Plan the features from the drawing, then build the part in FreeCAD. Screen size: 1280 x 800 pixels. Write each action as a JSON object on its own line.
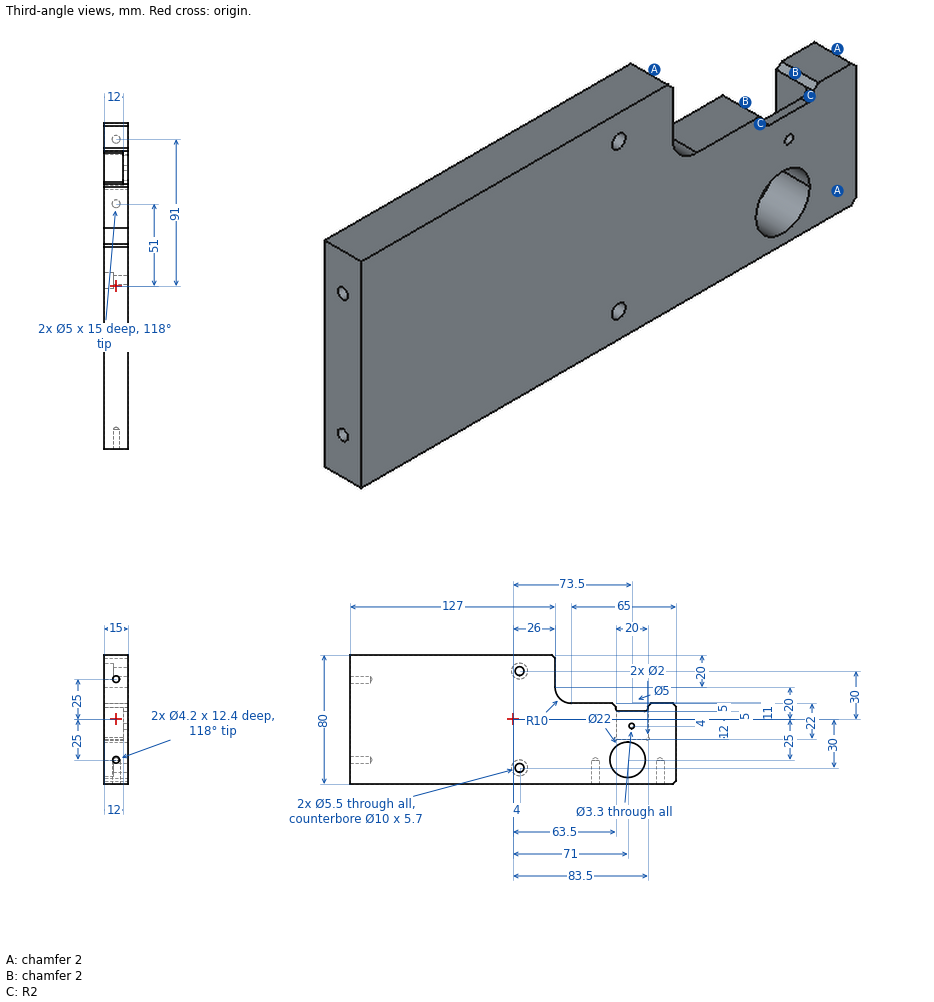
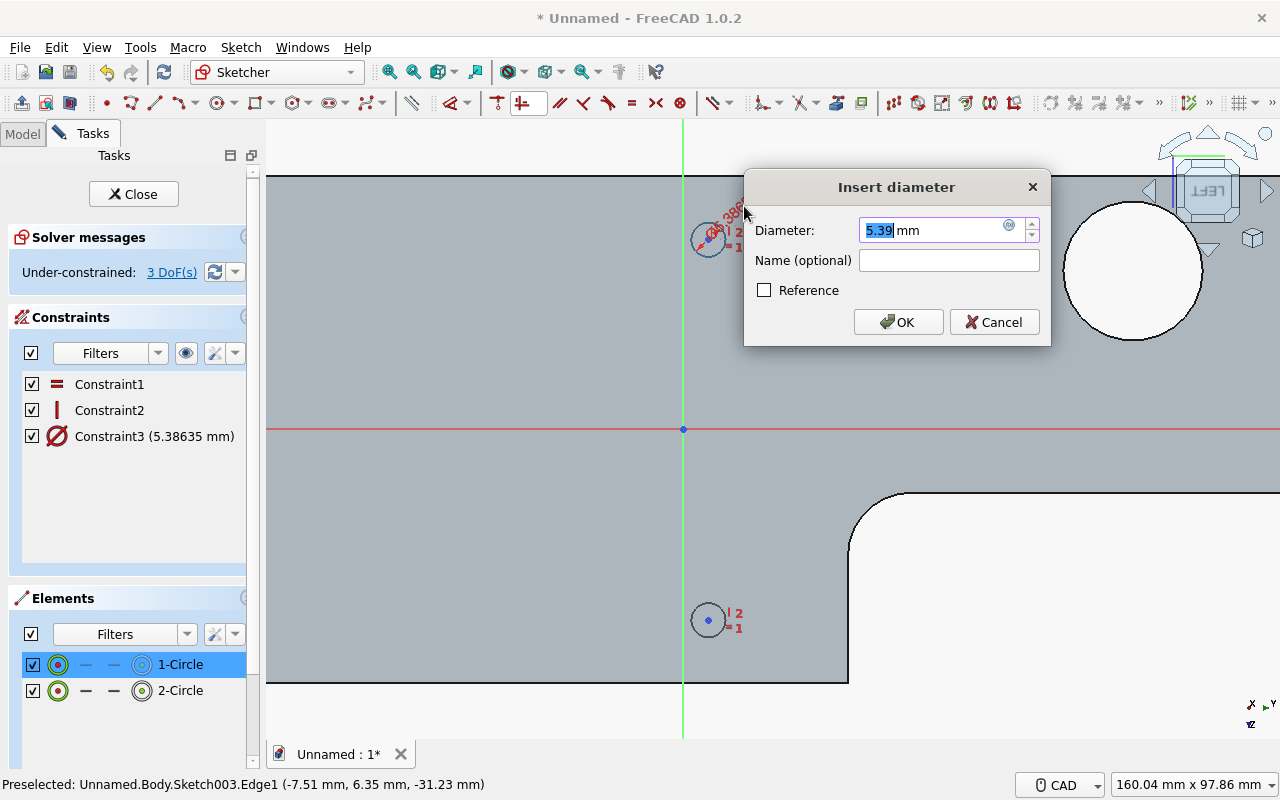
{"action": "type", "text": "5.5"}
{"action": "key", "text": "Return"}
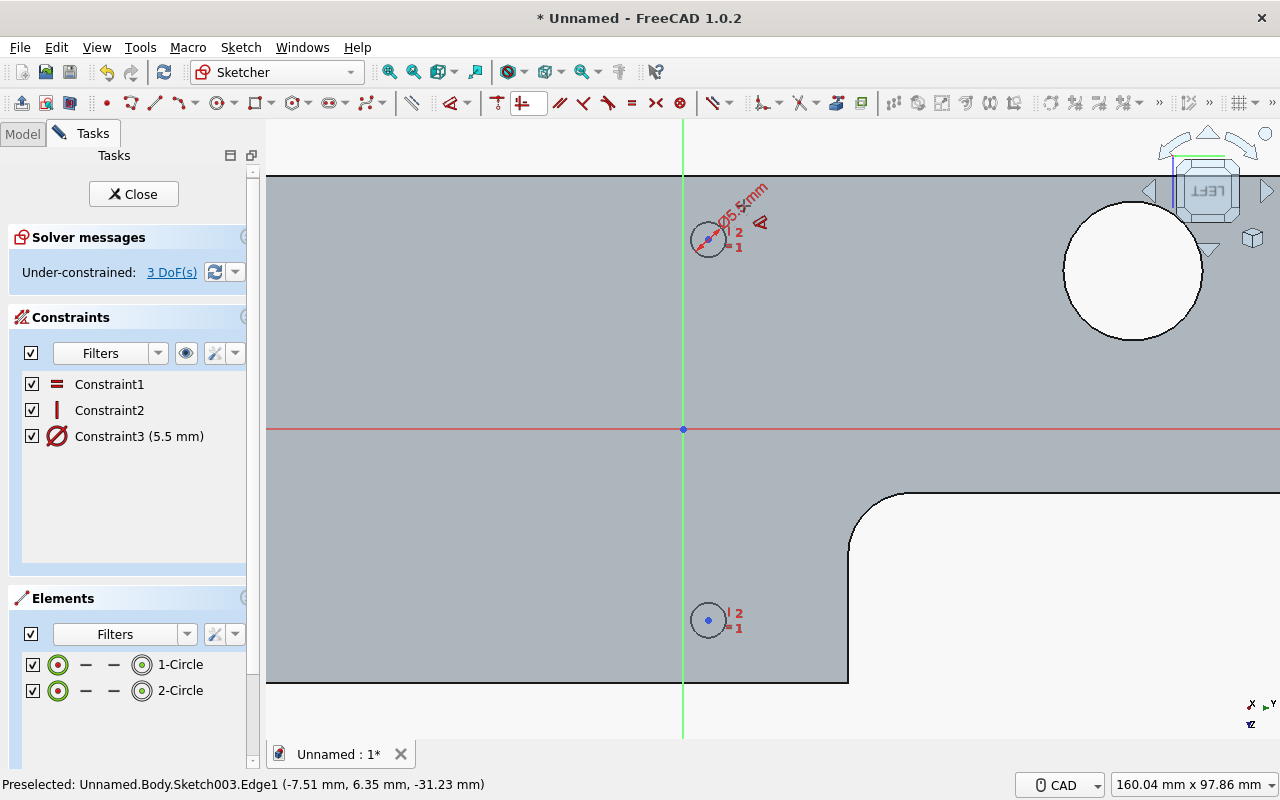
{"action": "scroll", "coordinate": [708, 240], "scroll_direction": "up", "scroll_amount": 3}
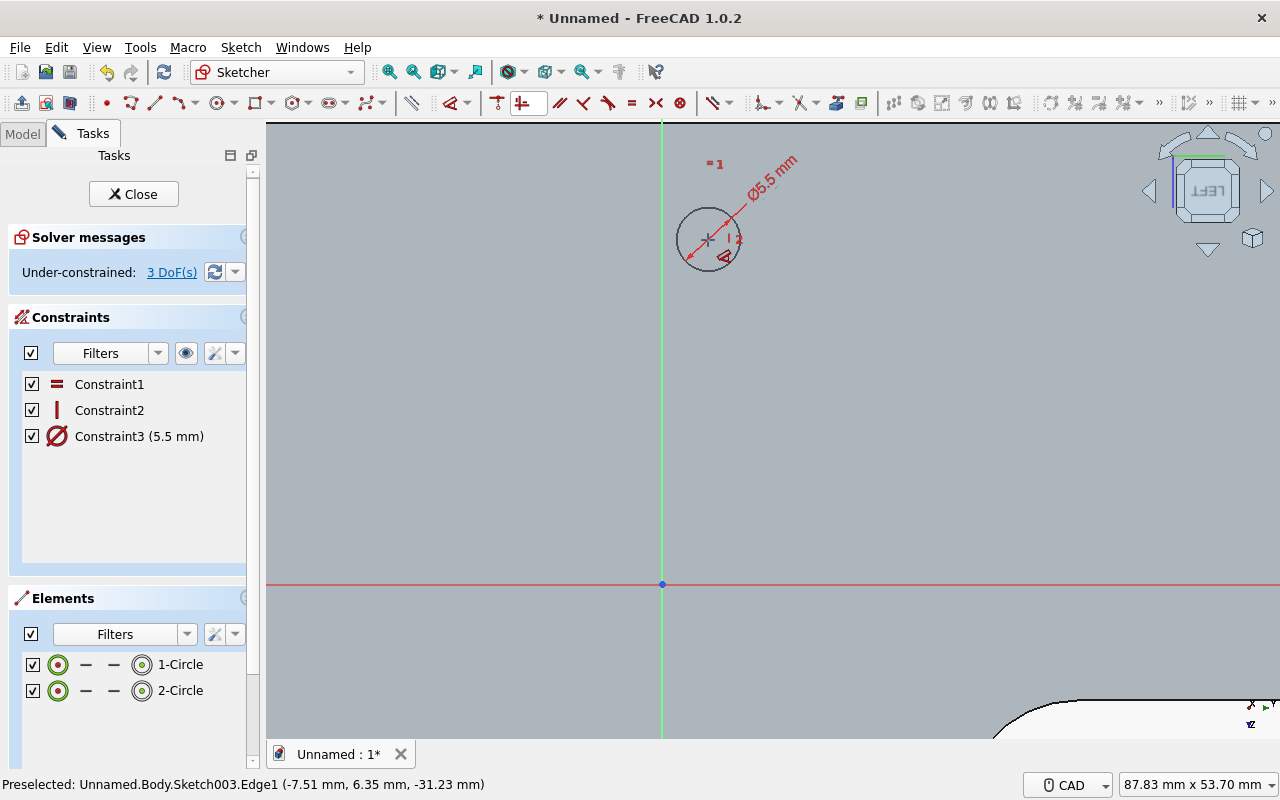
{"action": "left_click", "coordinate": [709, 239]}
{"action": "left_click", "coordinate": [685, 619]}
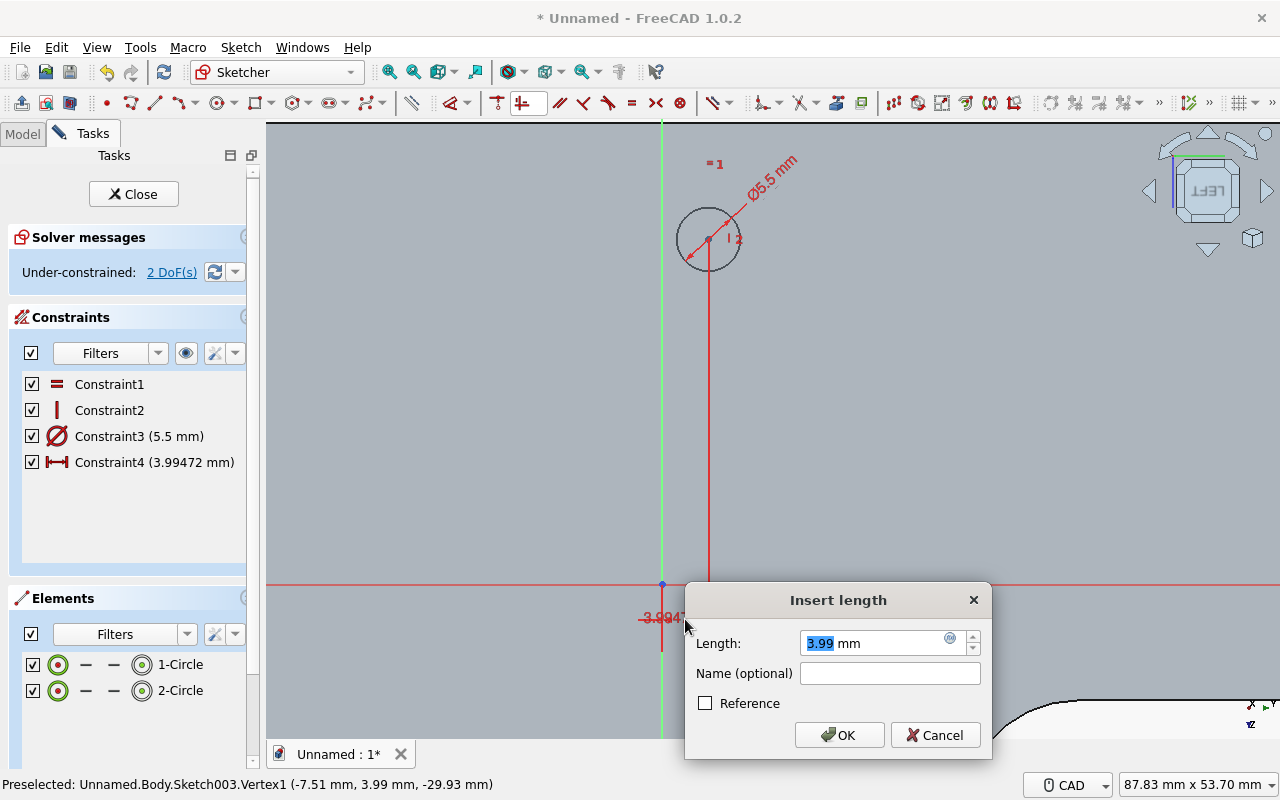
{"action": "type", "text": "4"}
{"action": "key", "text": "Return"}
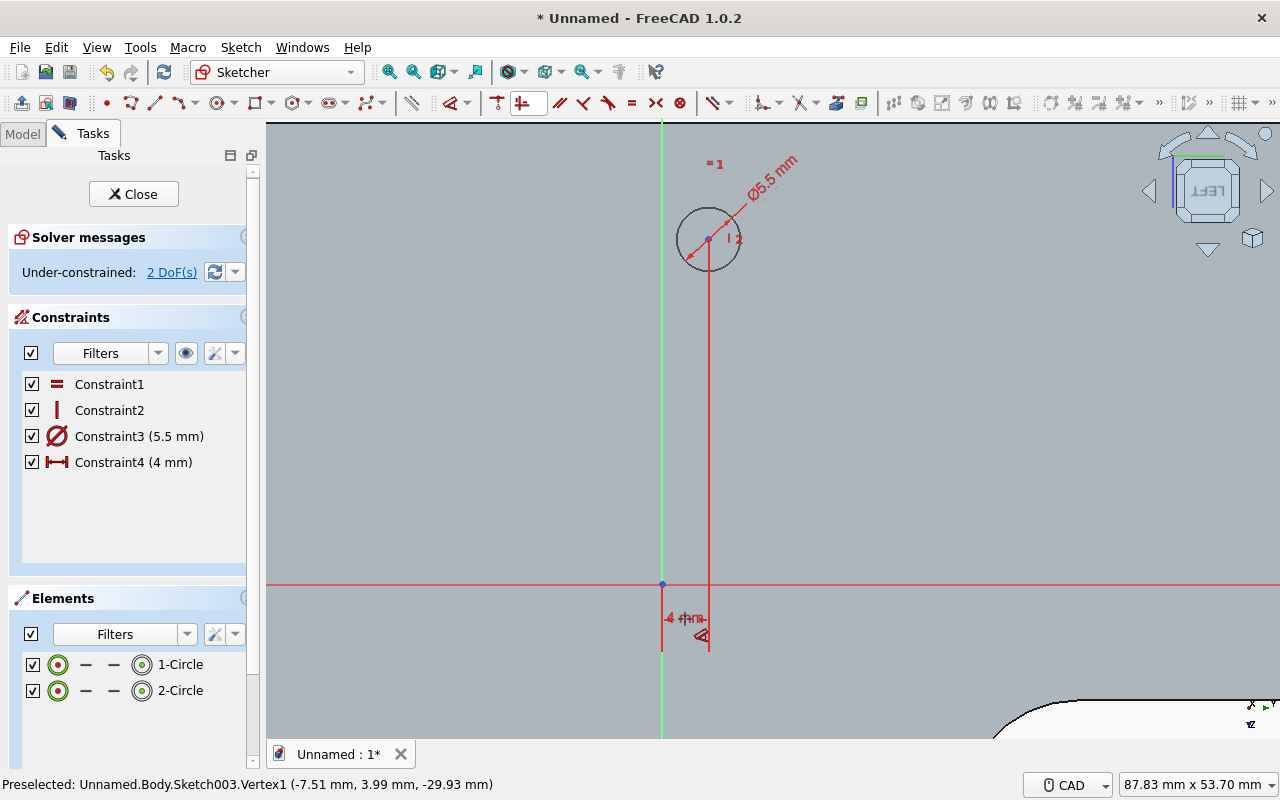
{"action": "left_click", "coordinate": [709, 239]}
{"action": "left_click", "coordinate": [628, 412]}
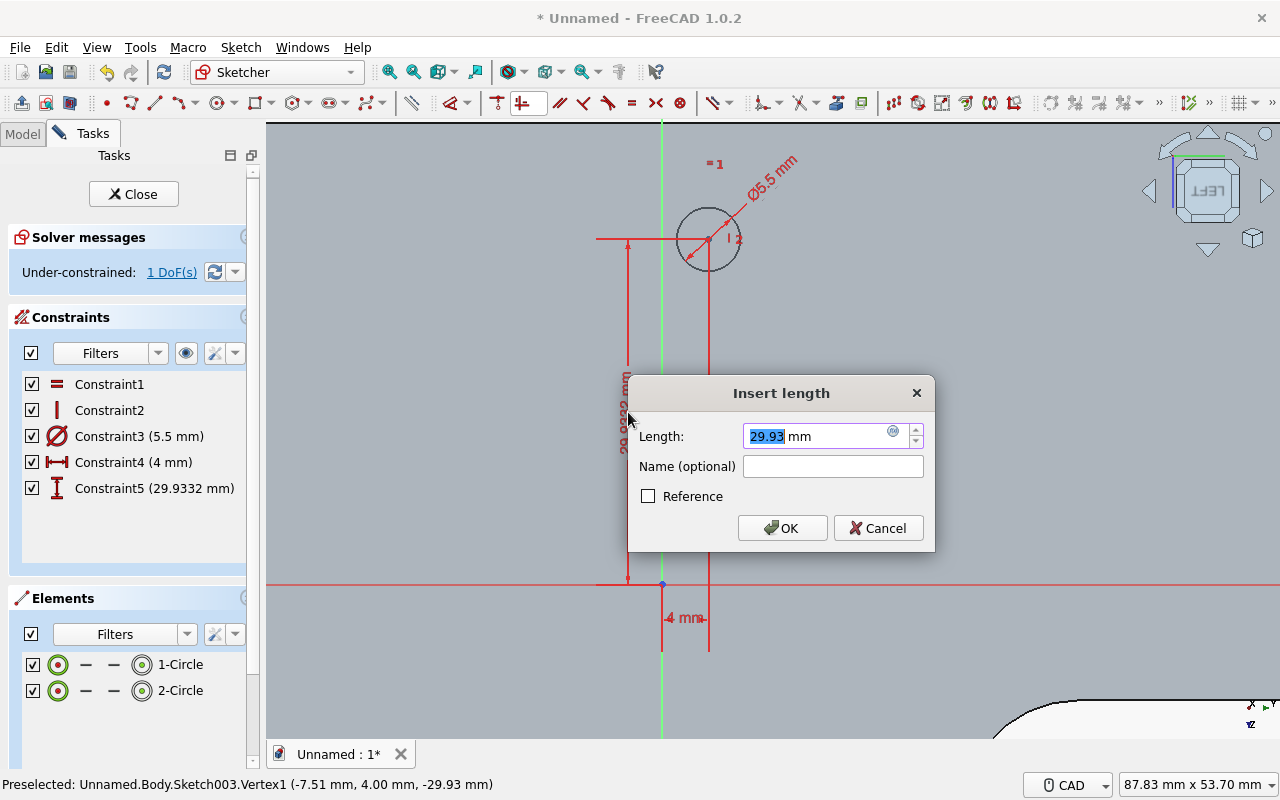
{"action": "type", "text": "30"}
{"action": "key", "text": "Return"}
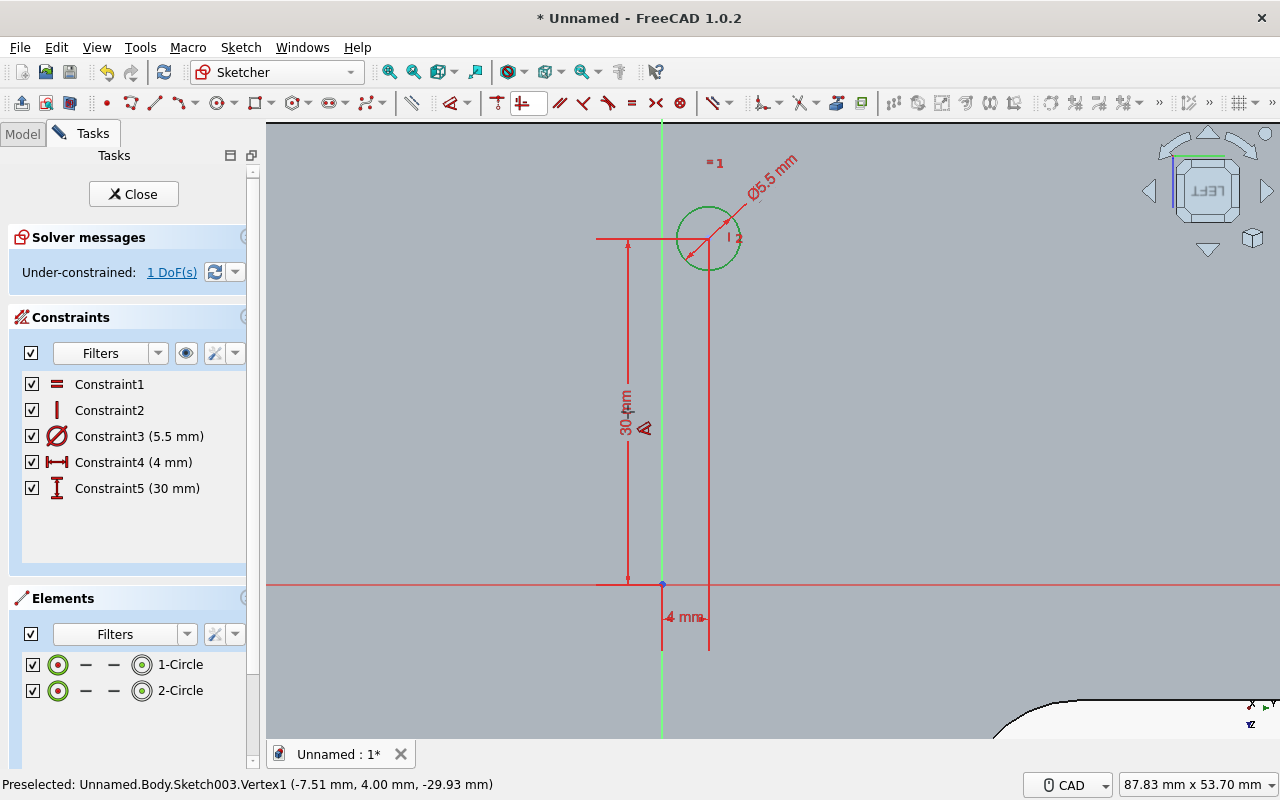
{"action": "scroll", "coordinate": [708, 239], "scroll_direction": "down", "scroll_amount": 3}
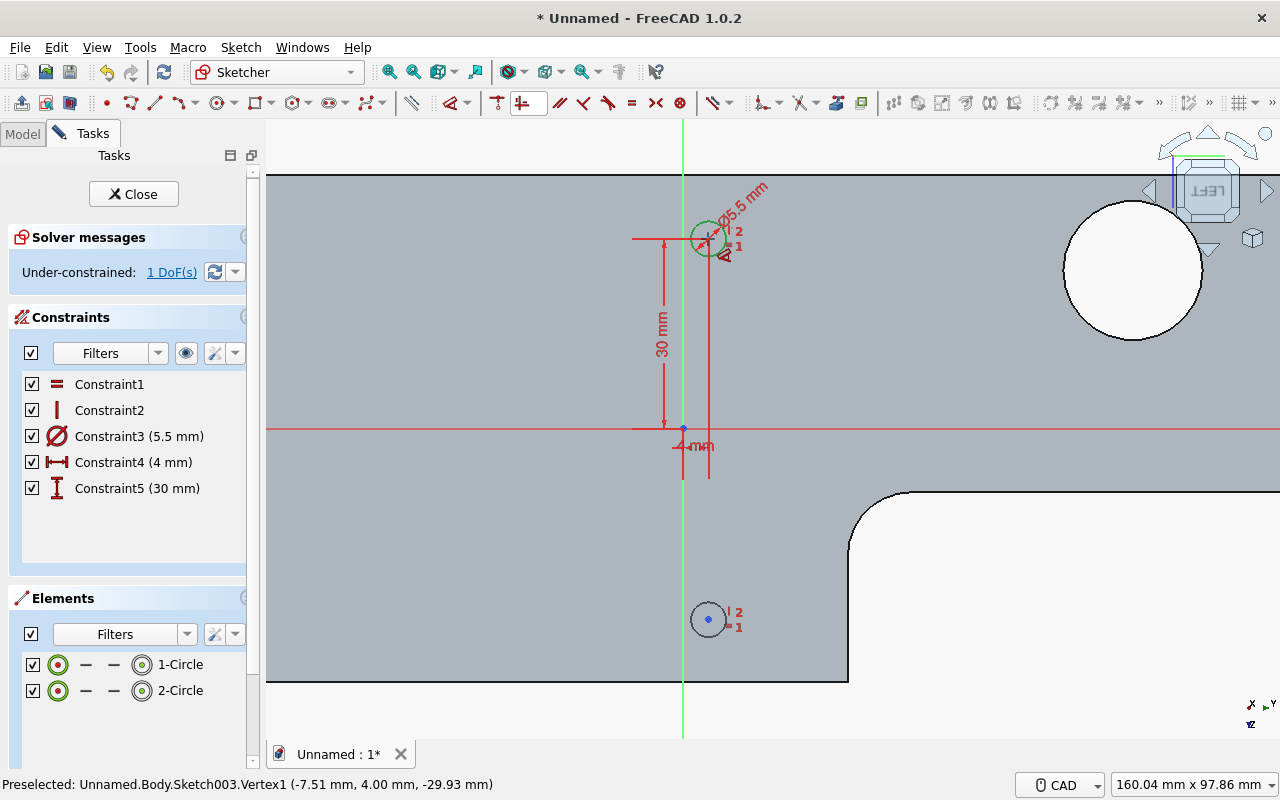
{"action": "left_click", "coordinate": [709, 620]}
{"action": "left_click", "coordinate": [649, 524]}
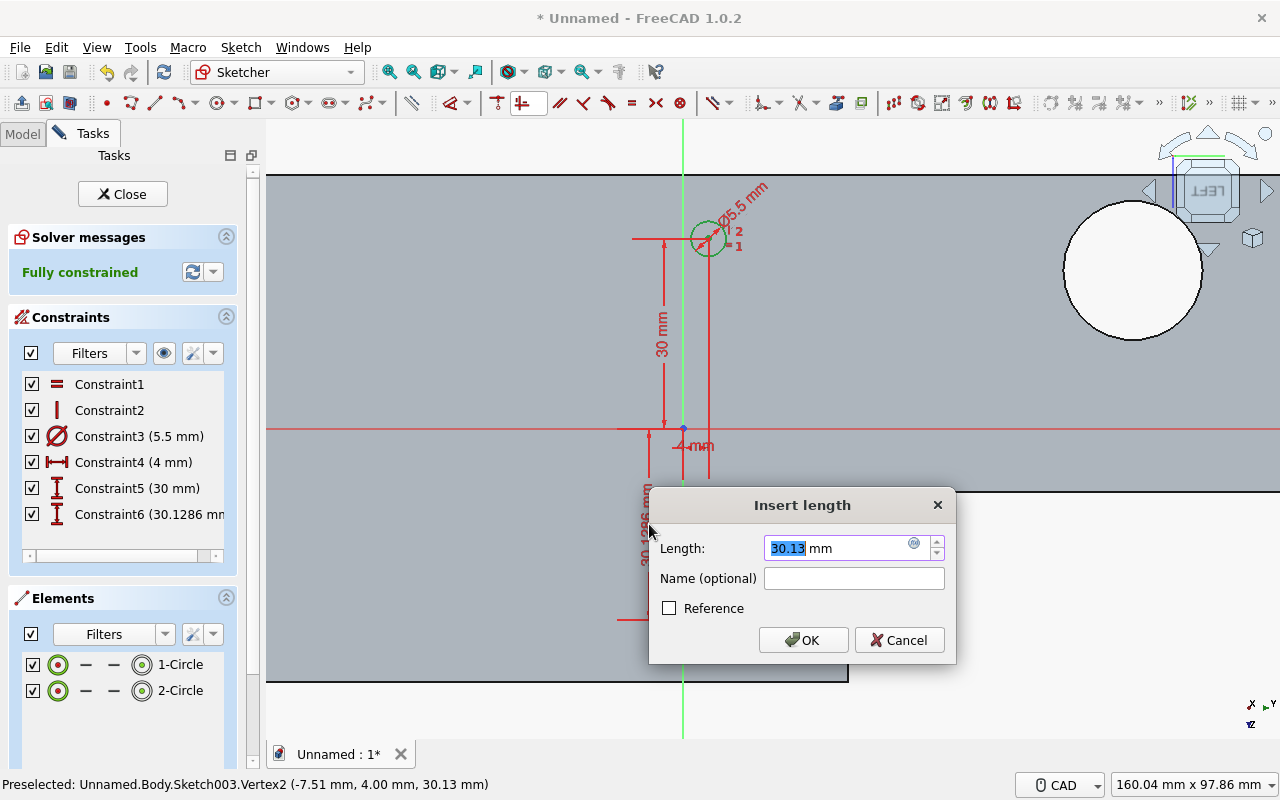
{"action": "type", "text": "30"}
{"action": "key", "text": "Return"}
{"action": "key", "text": "Escape"}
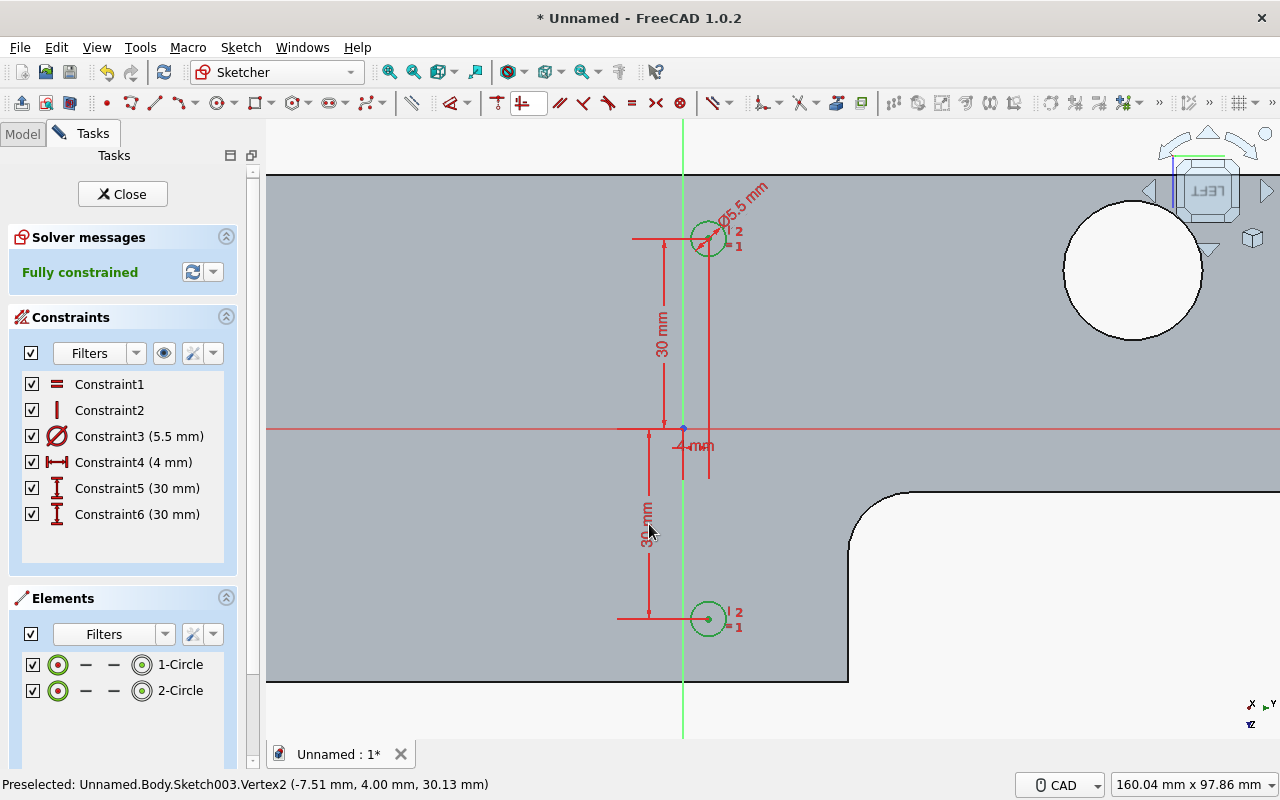
{"action": "left_click", "coordinate": [123, 194]}